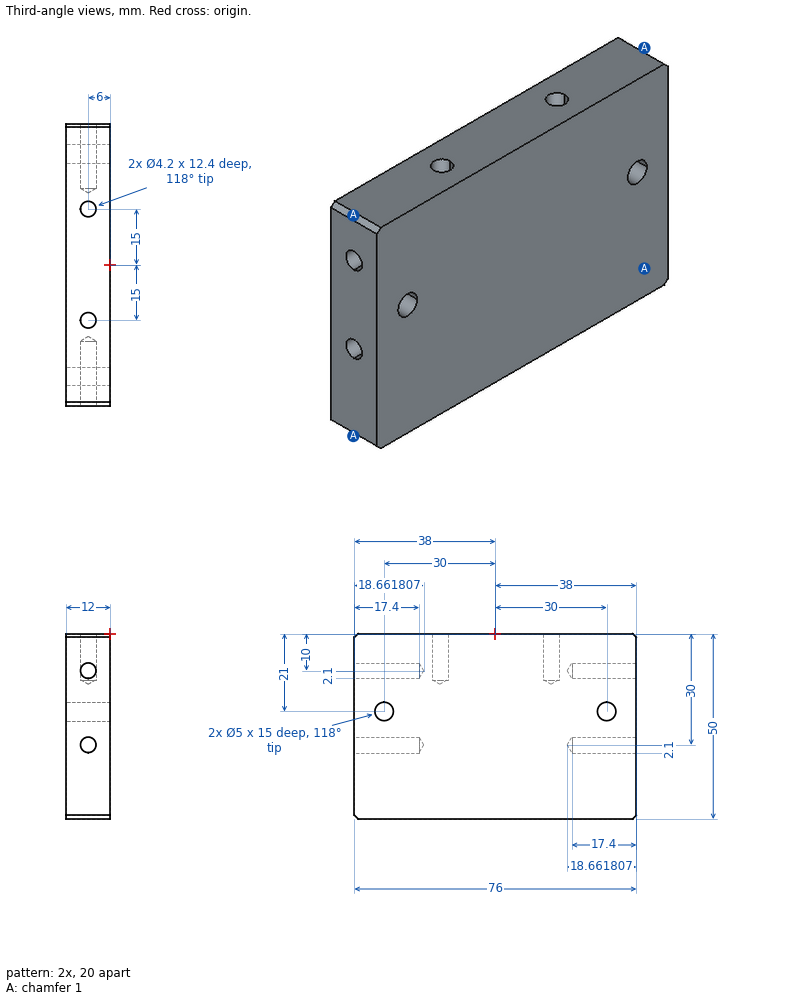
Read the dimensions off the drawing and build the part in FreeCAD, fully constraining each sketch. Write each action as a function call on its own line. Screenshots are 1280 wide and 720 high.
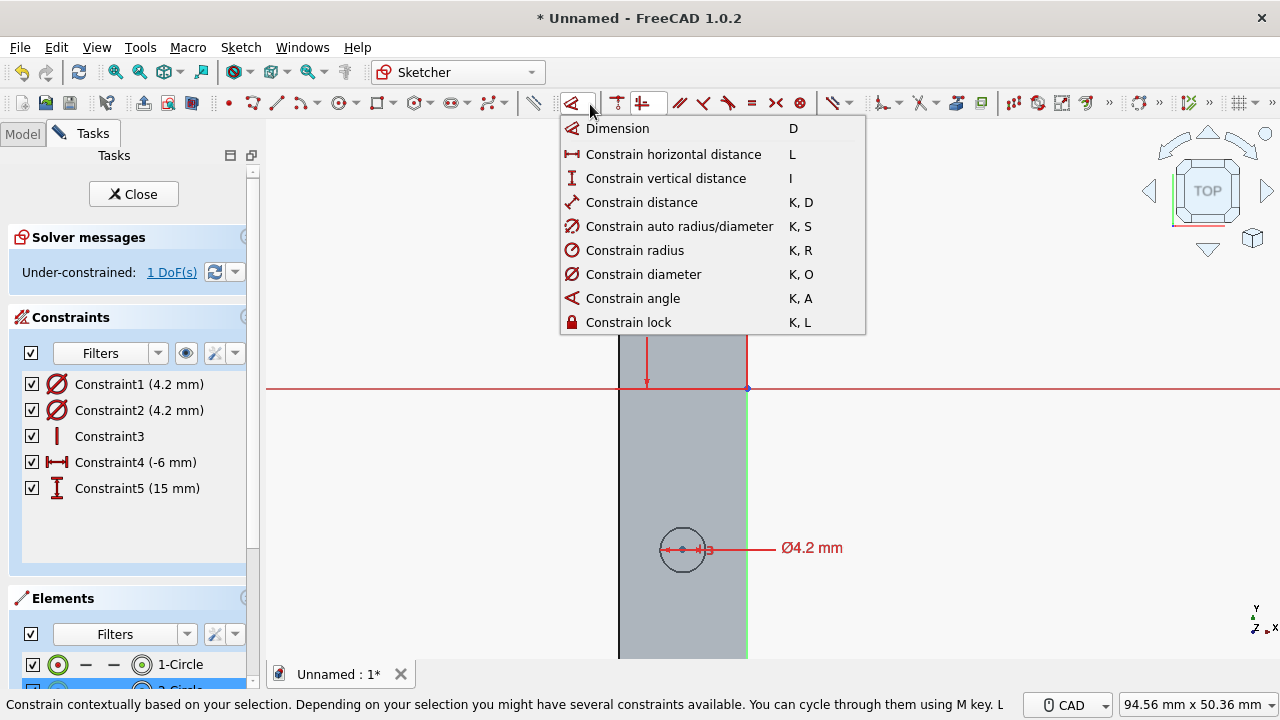
click(713, 178)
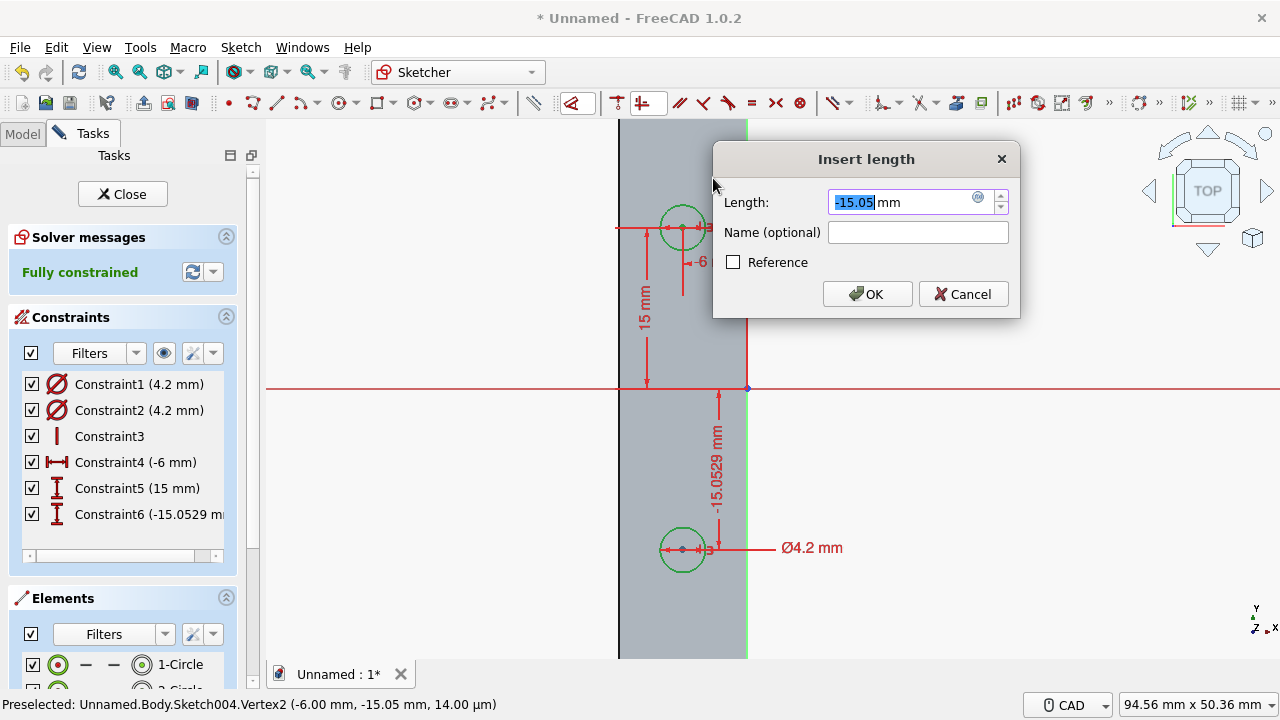
text(-15)
key(Return)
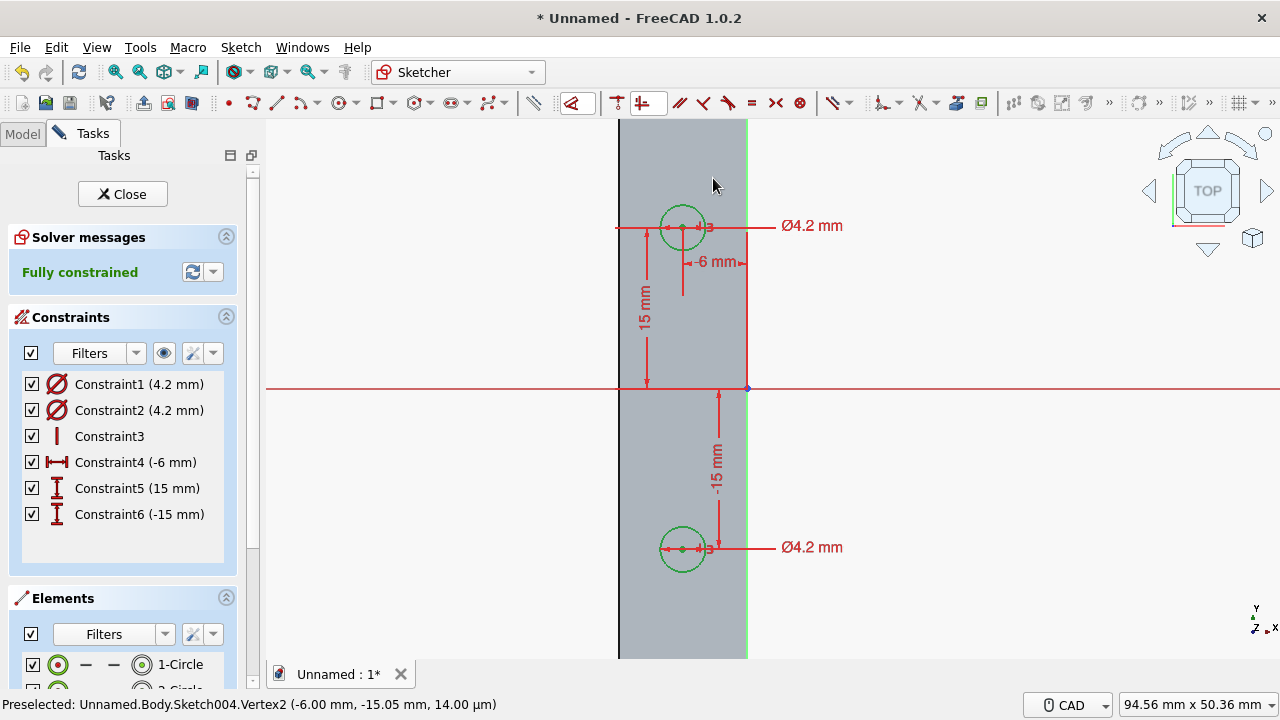
click(123, 194)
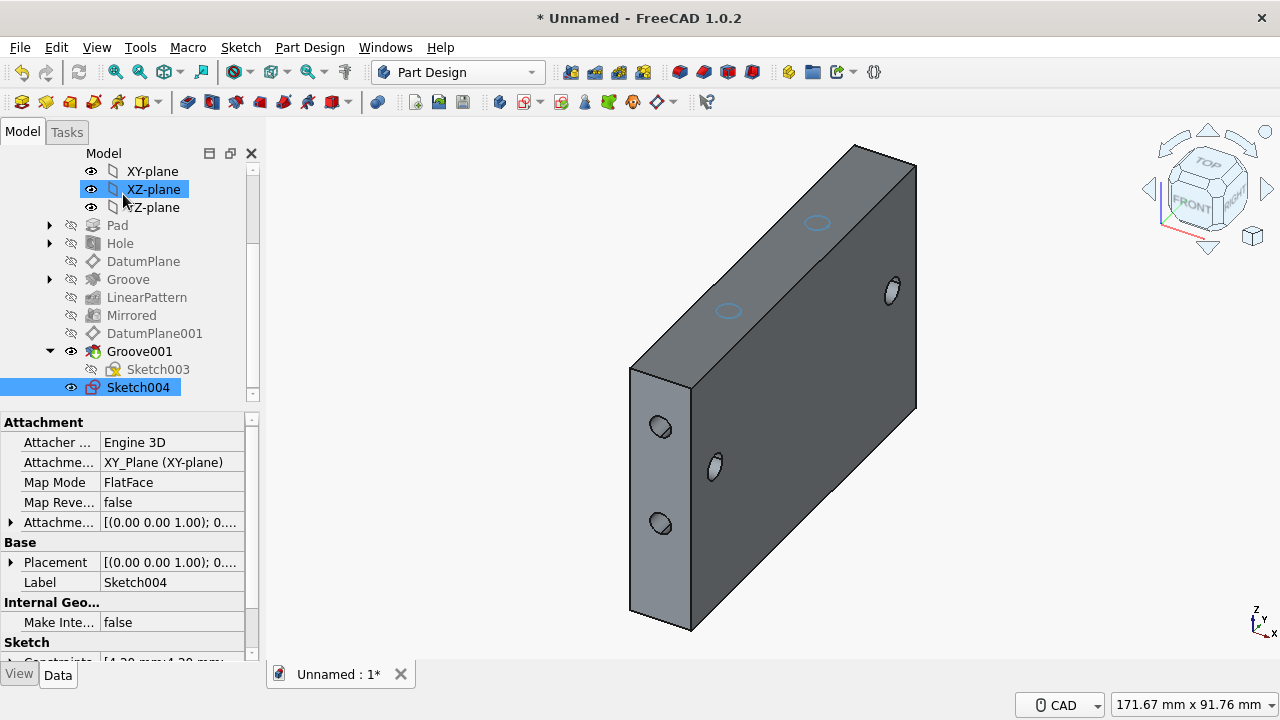
click(212, 102)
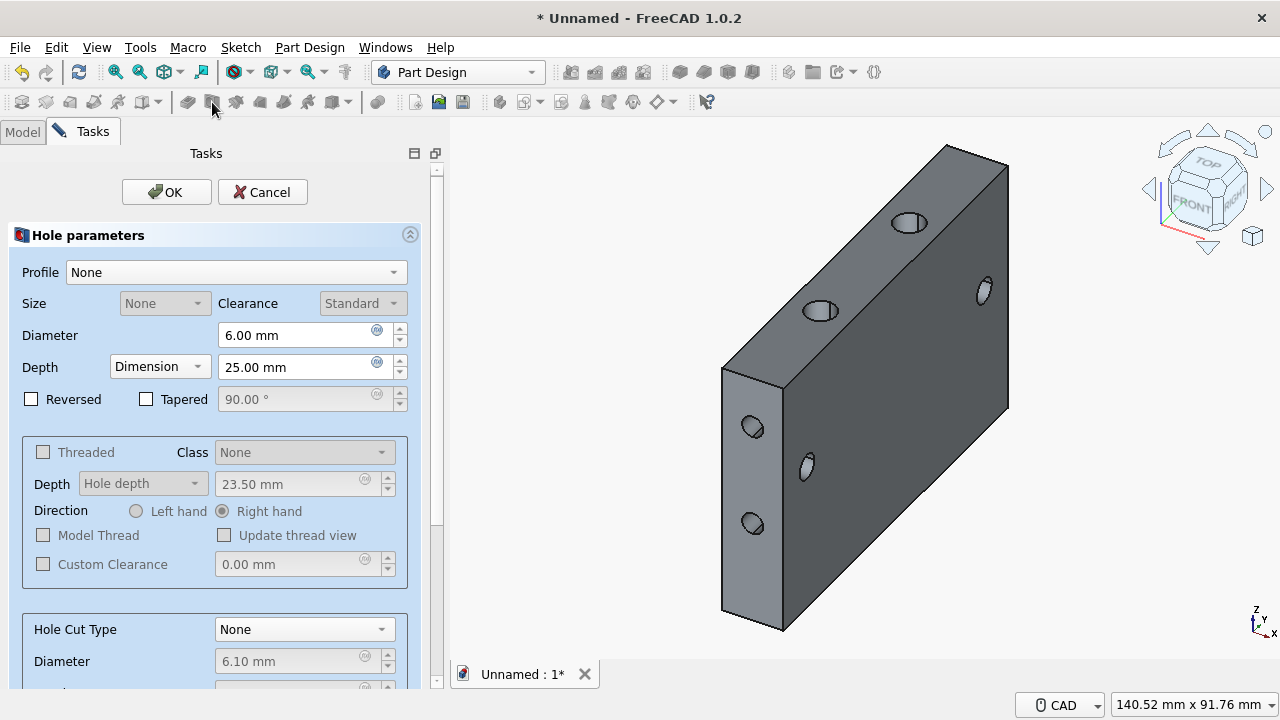
triple_click(305, 335)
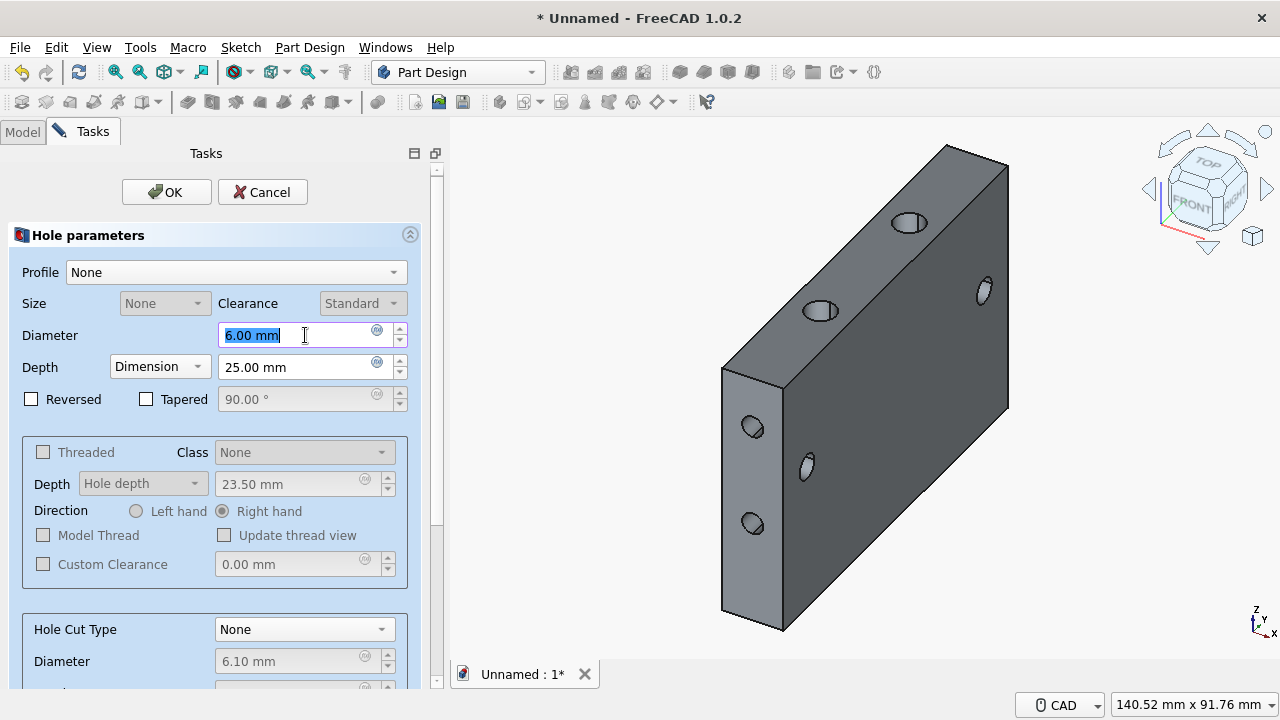
text(4.2)
key(Tab)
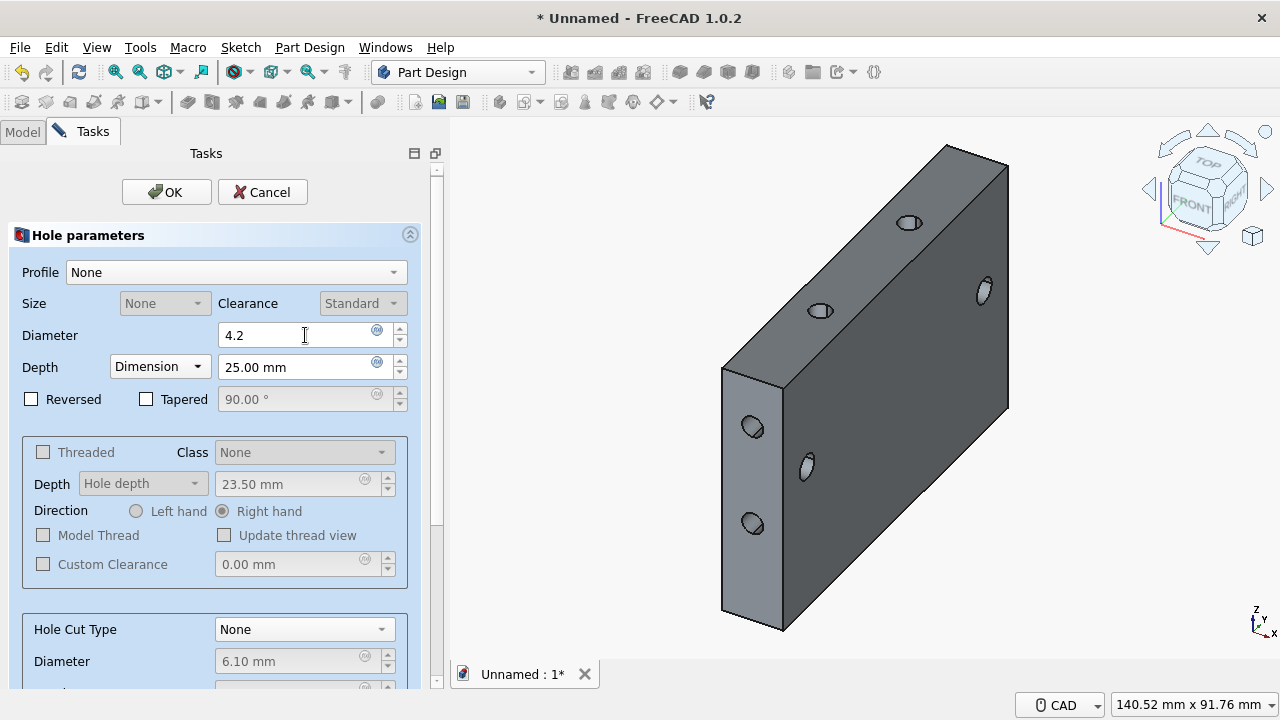
triple_click(305, 367)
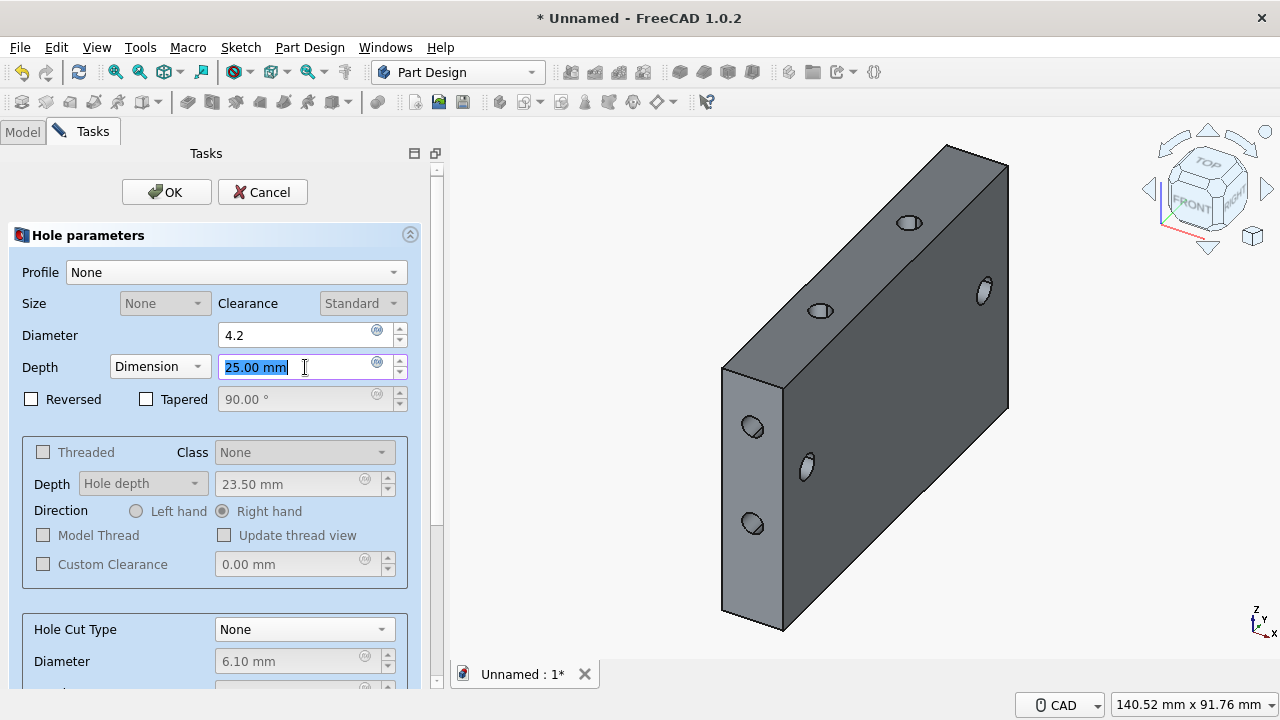
text(12.4)
key(Tab)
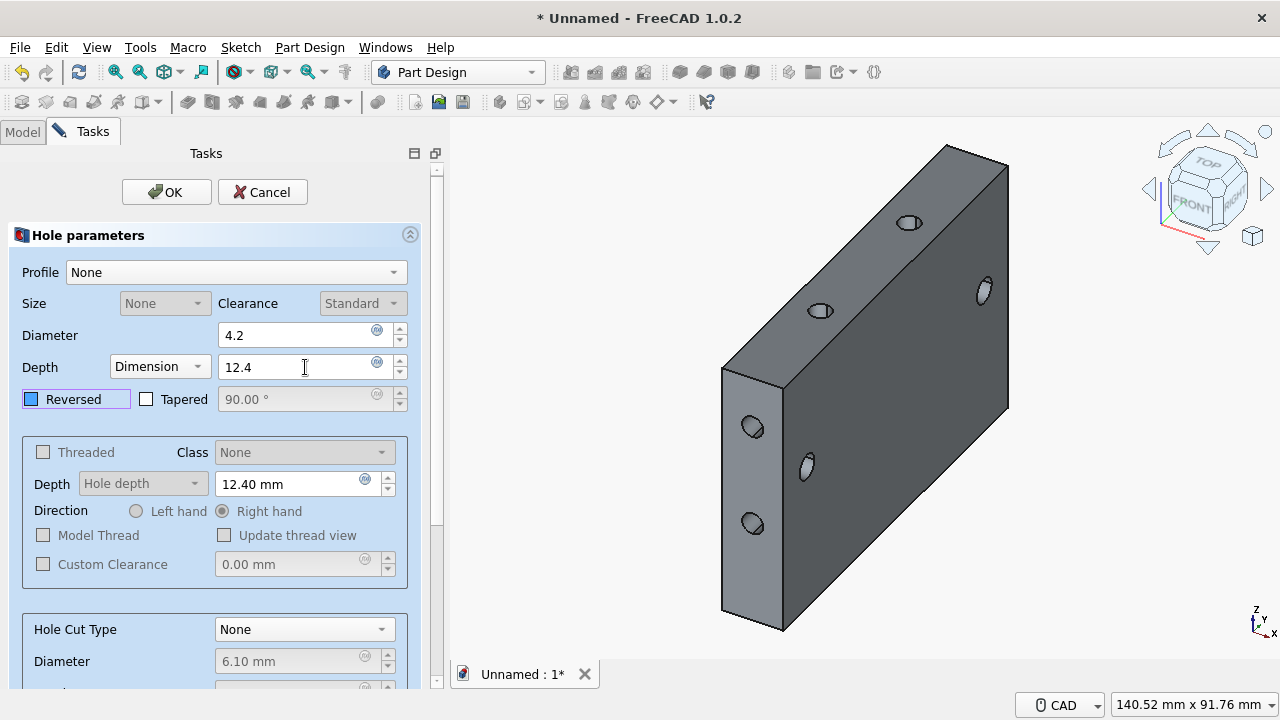
click(167, 192)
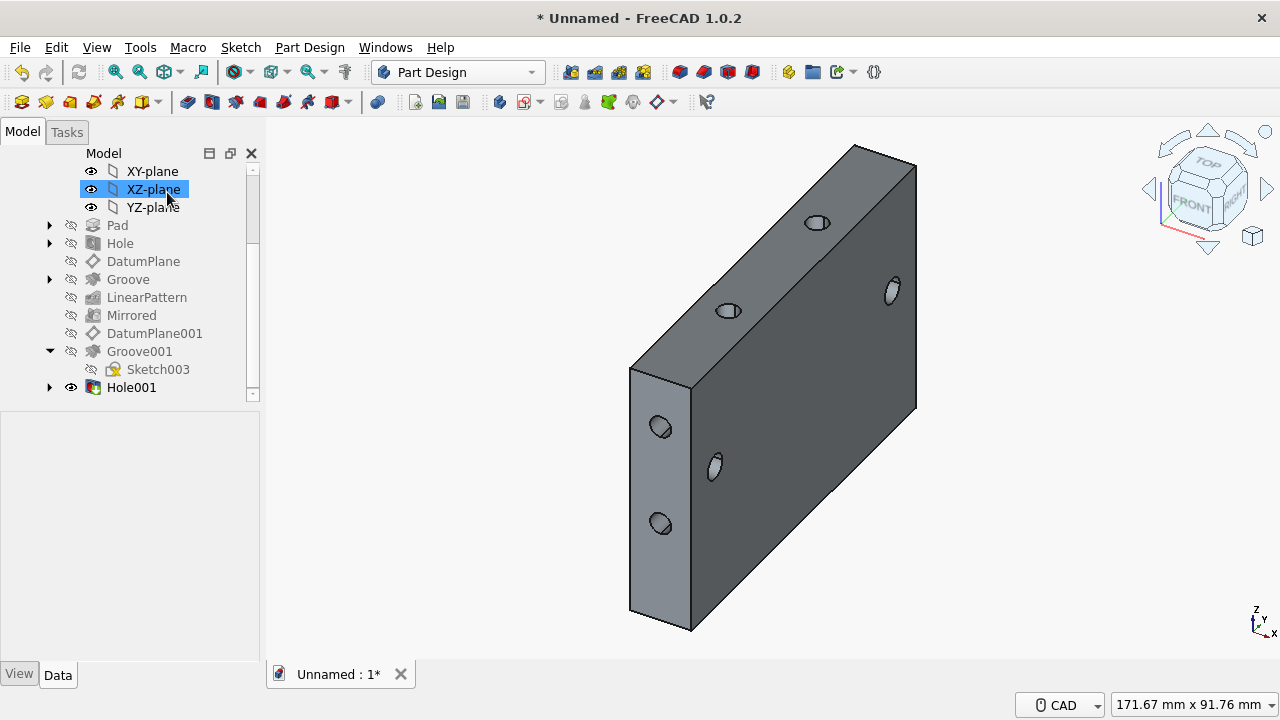
click(661, 378)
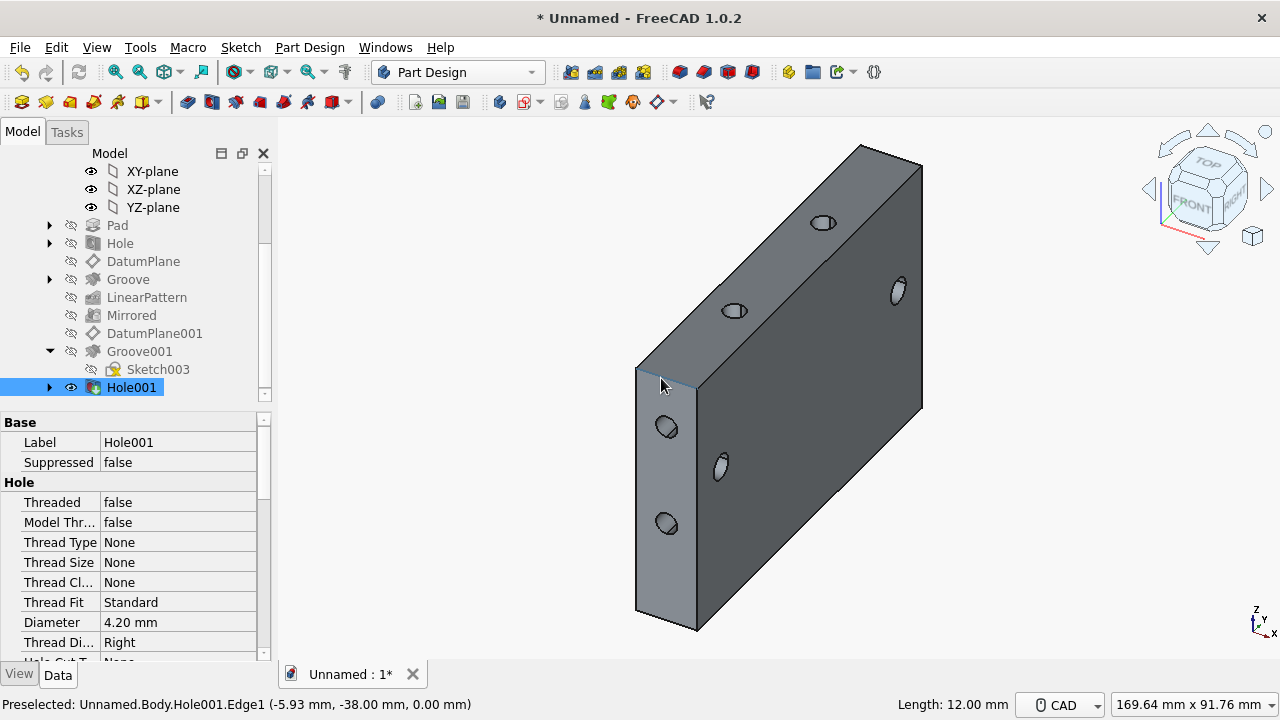
key(0)